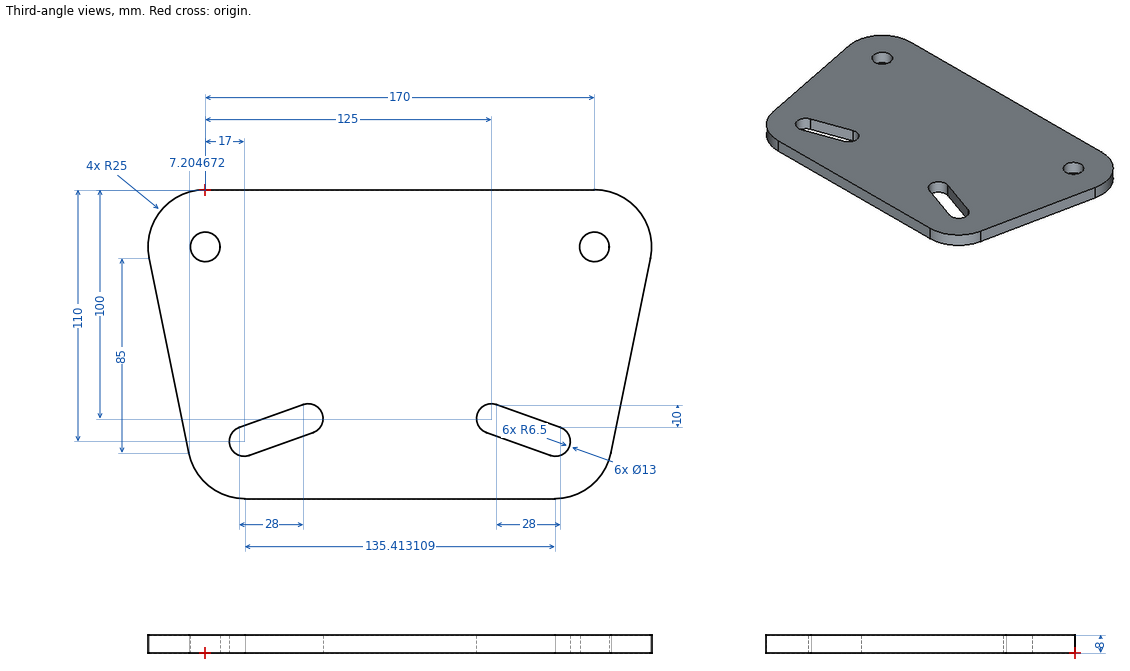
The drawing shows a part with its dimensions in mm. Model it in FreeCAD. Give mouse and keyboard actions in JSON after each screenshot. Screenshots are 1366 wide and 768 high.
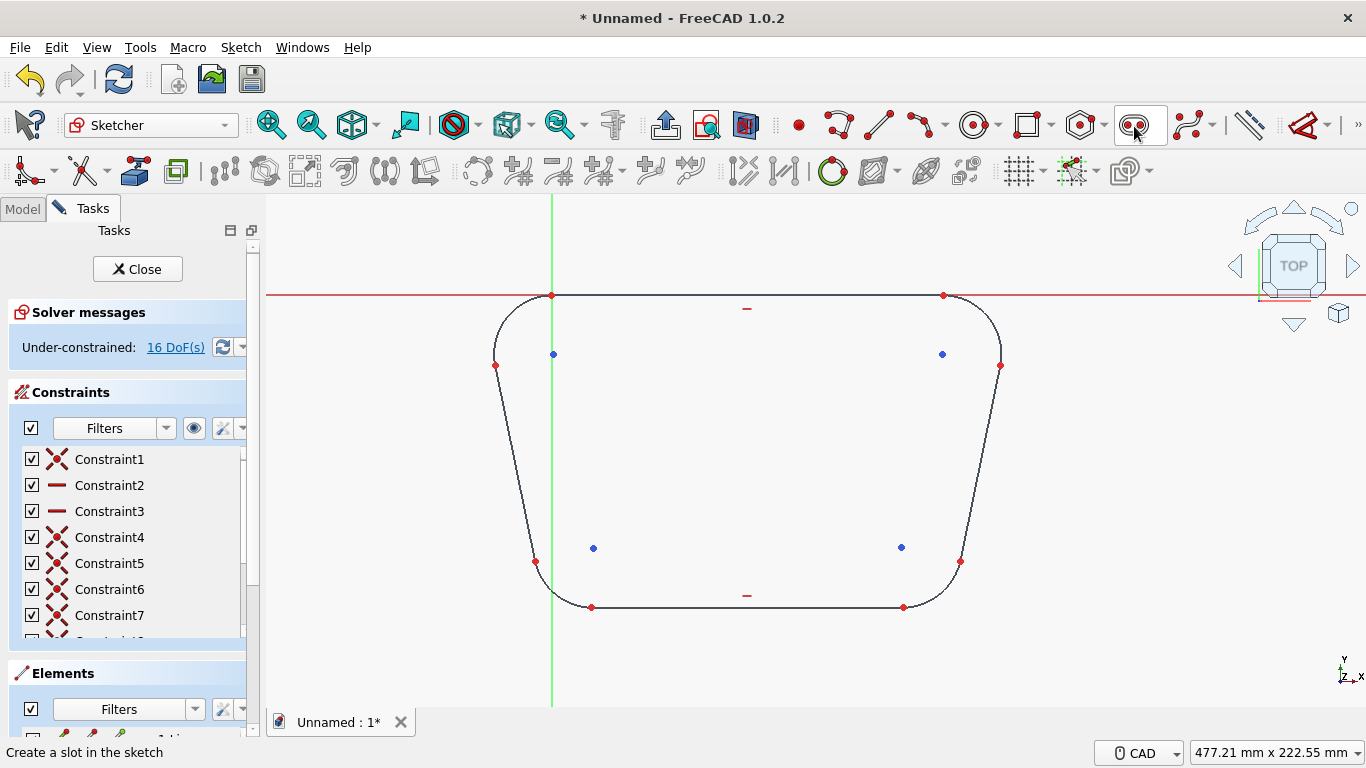
{"action": "scroll", "coordinate": [840, 526], "scroll_direction": "up", "scroll_amount": 3}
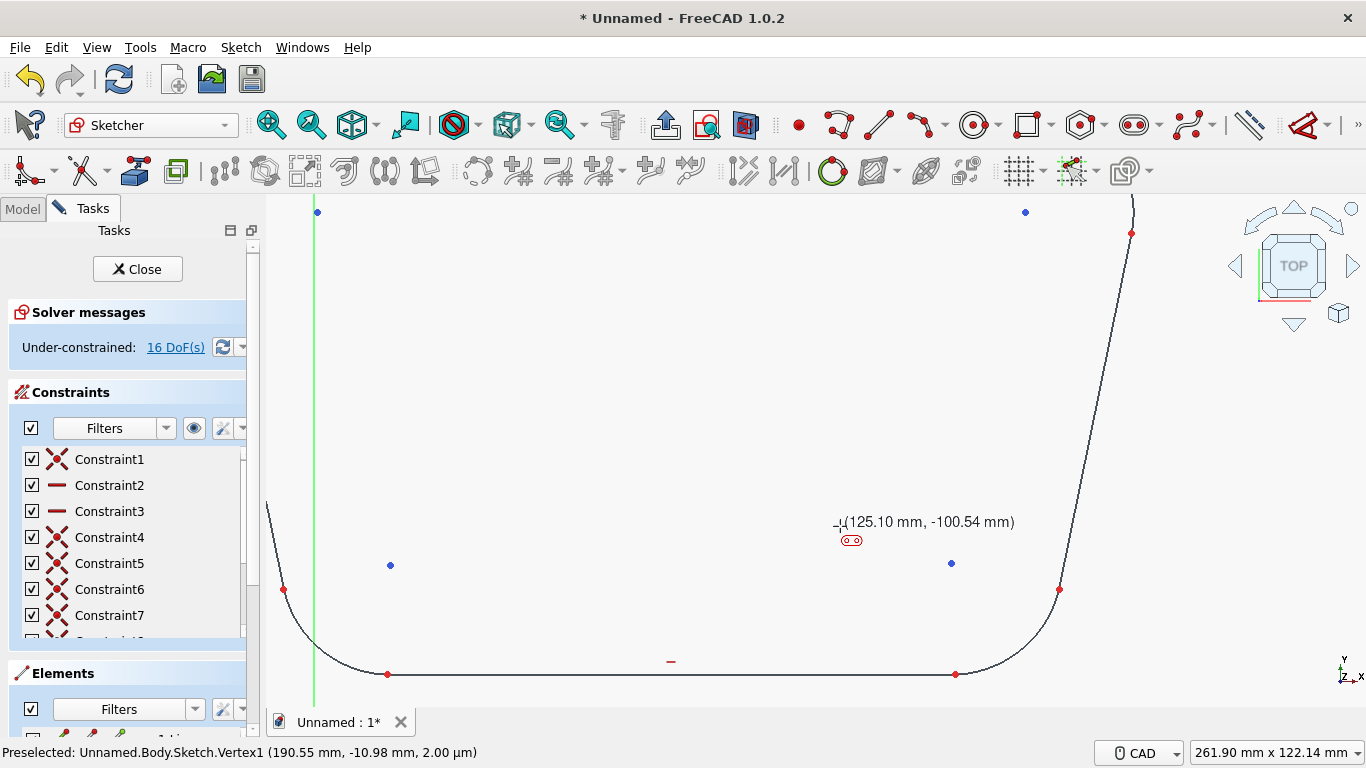
{"action": "left_click", "coordinate": [839, 525]}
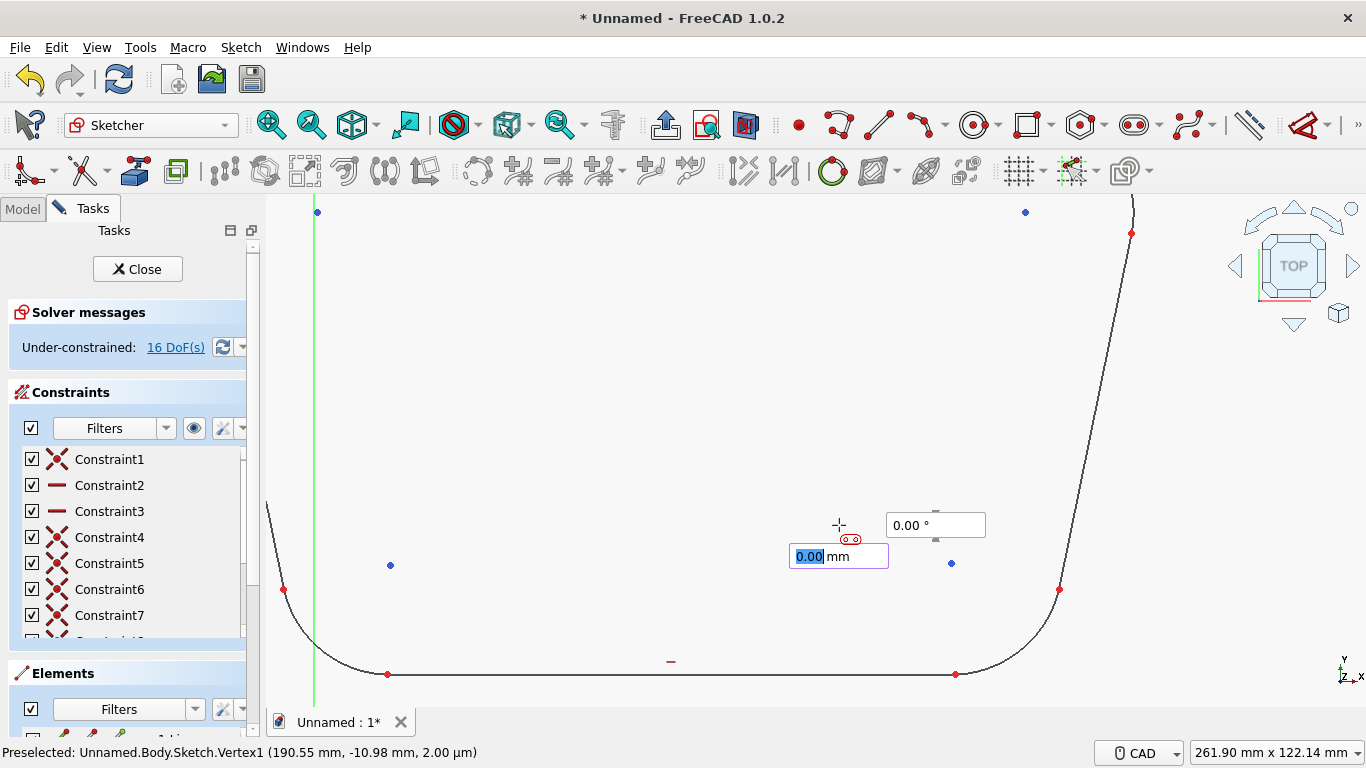
{"action": "scroll", "coordinate": [957, 567], "scroll_direction": "up", "scroll_amount": 13}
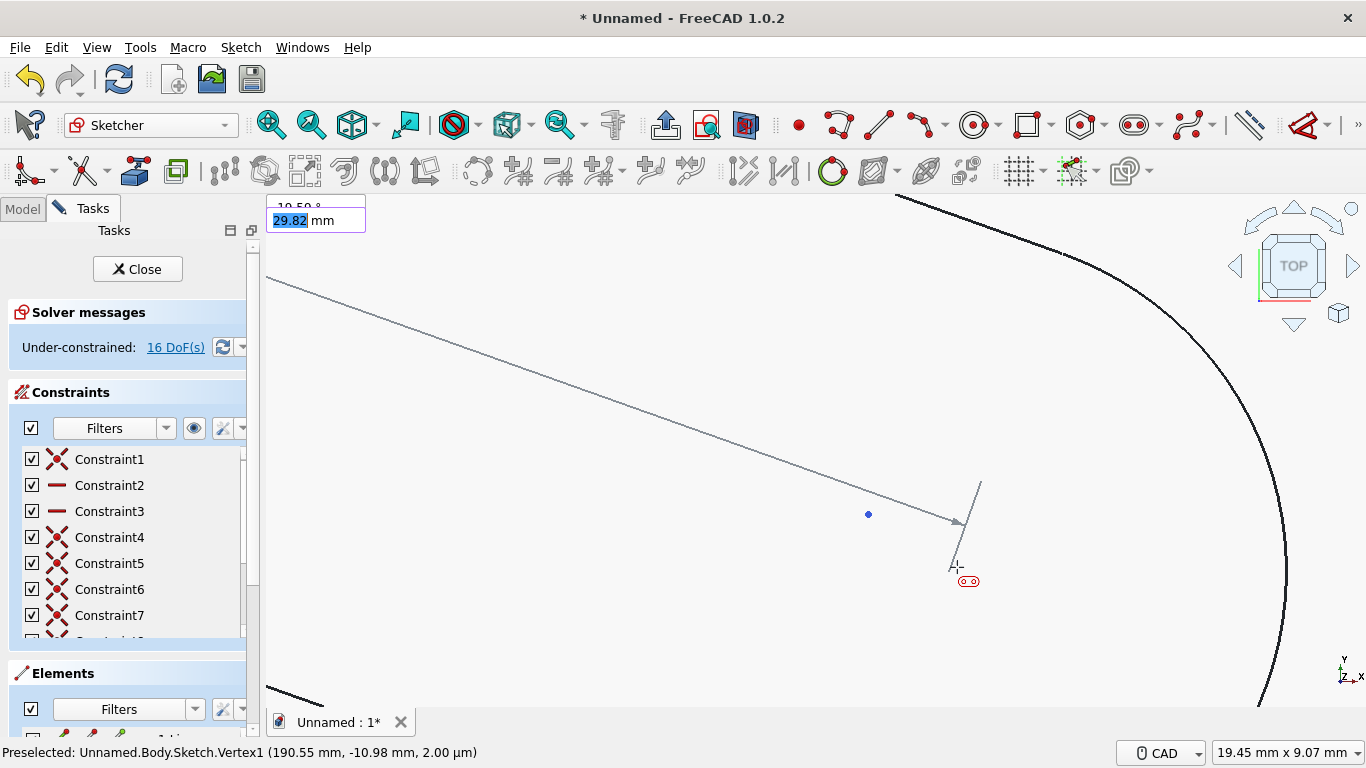
{"action": "left_click", "coordinate": [946, 558]}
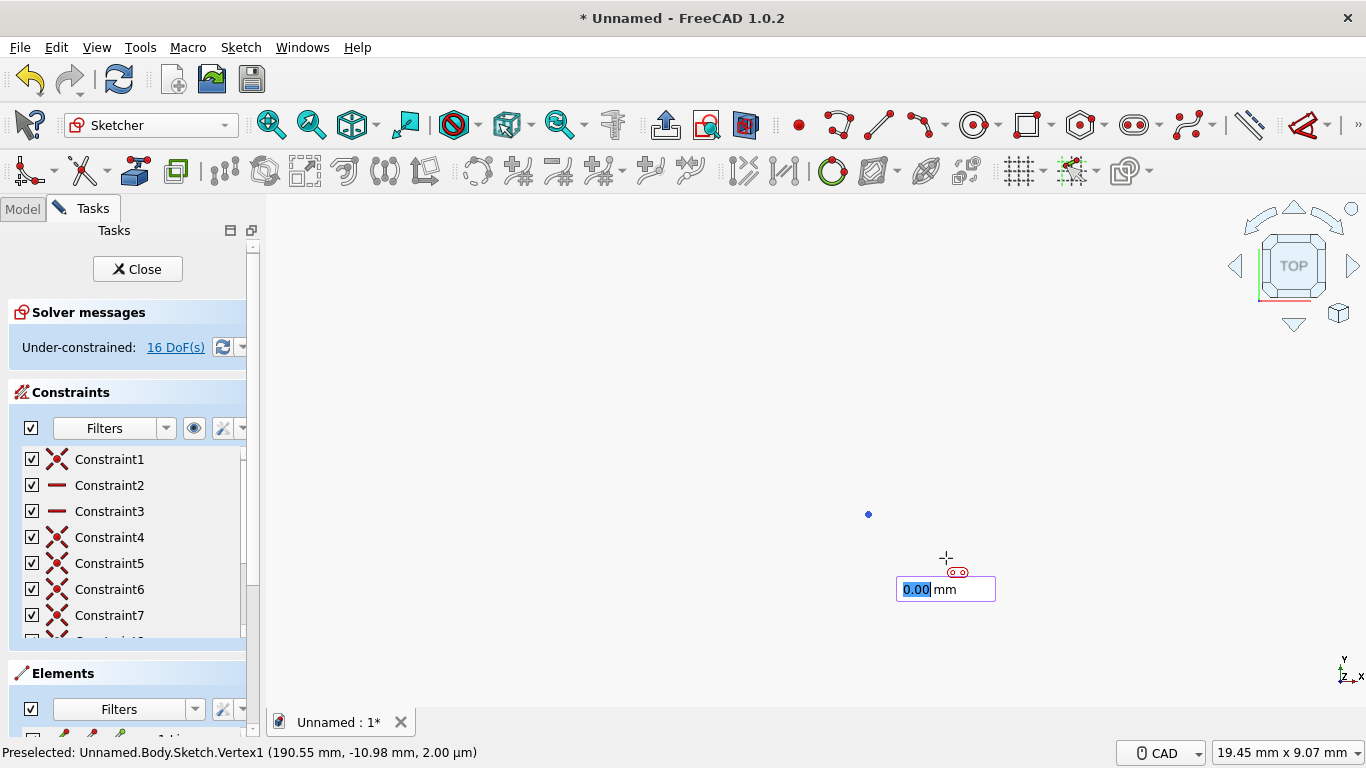
{"action": "scroll", "coordinate": [939, 571], "scroll_direction": "down", "scroll_amount": 15}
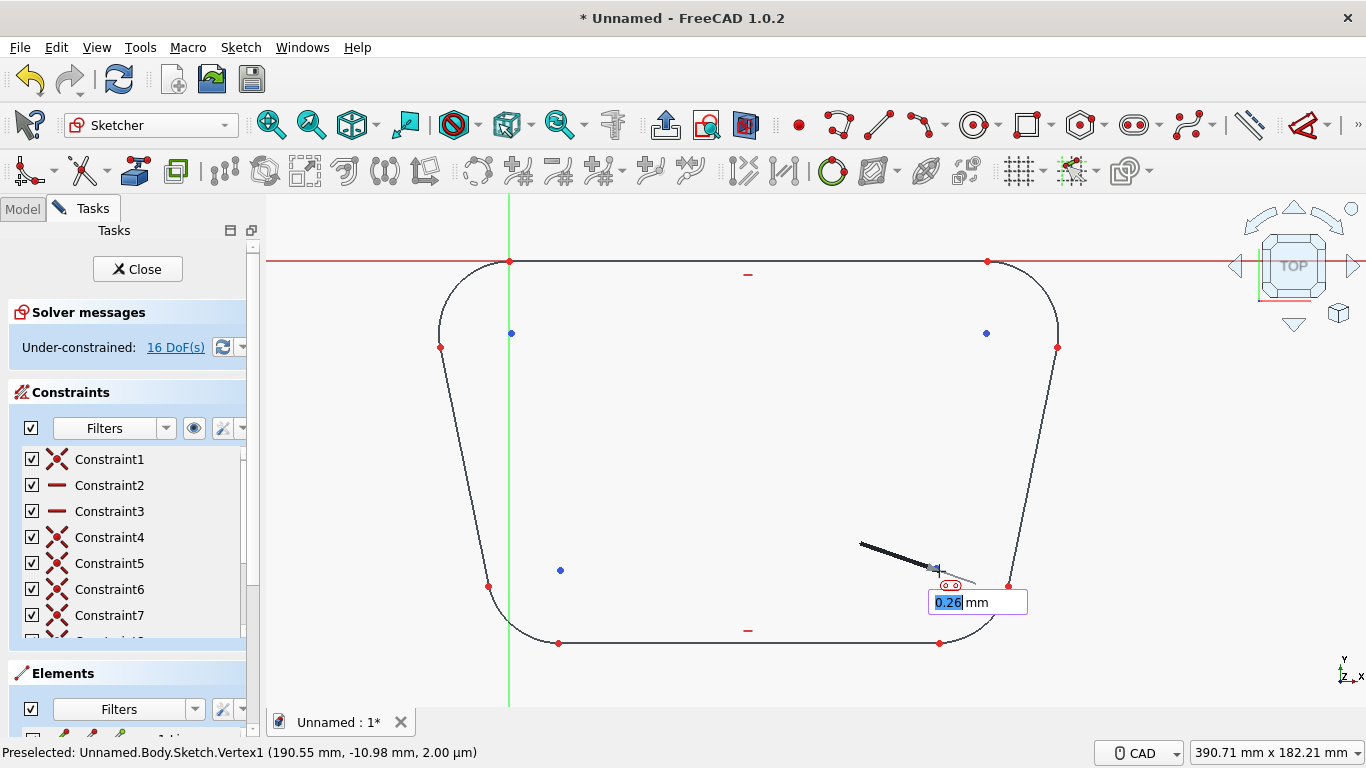
{"action": "left_click", "coordinate": [907, 540]}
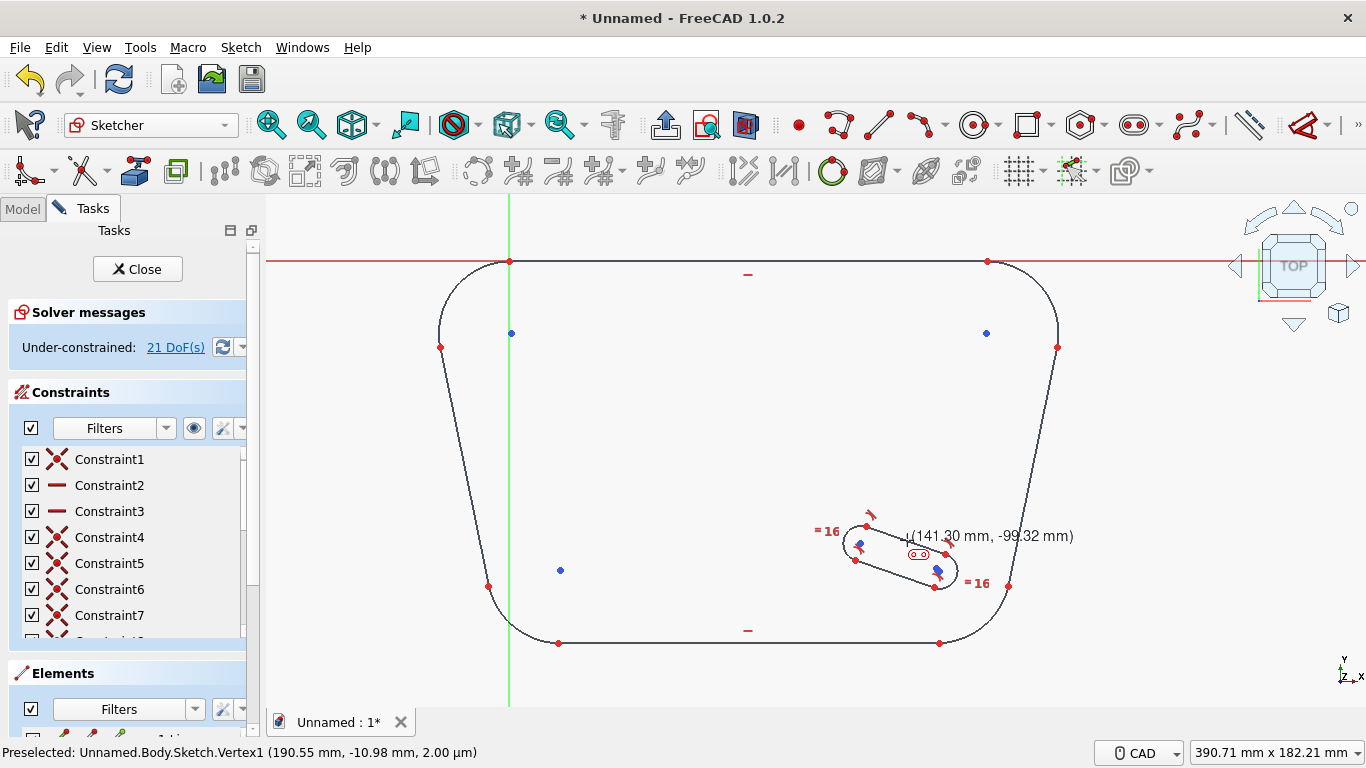
{"action": "scroll", "coordinate": [557, 571], "scroll_direction": "up", "scroll_amount": 15}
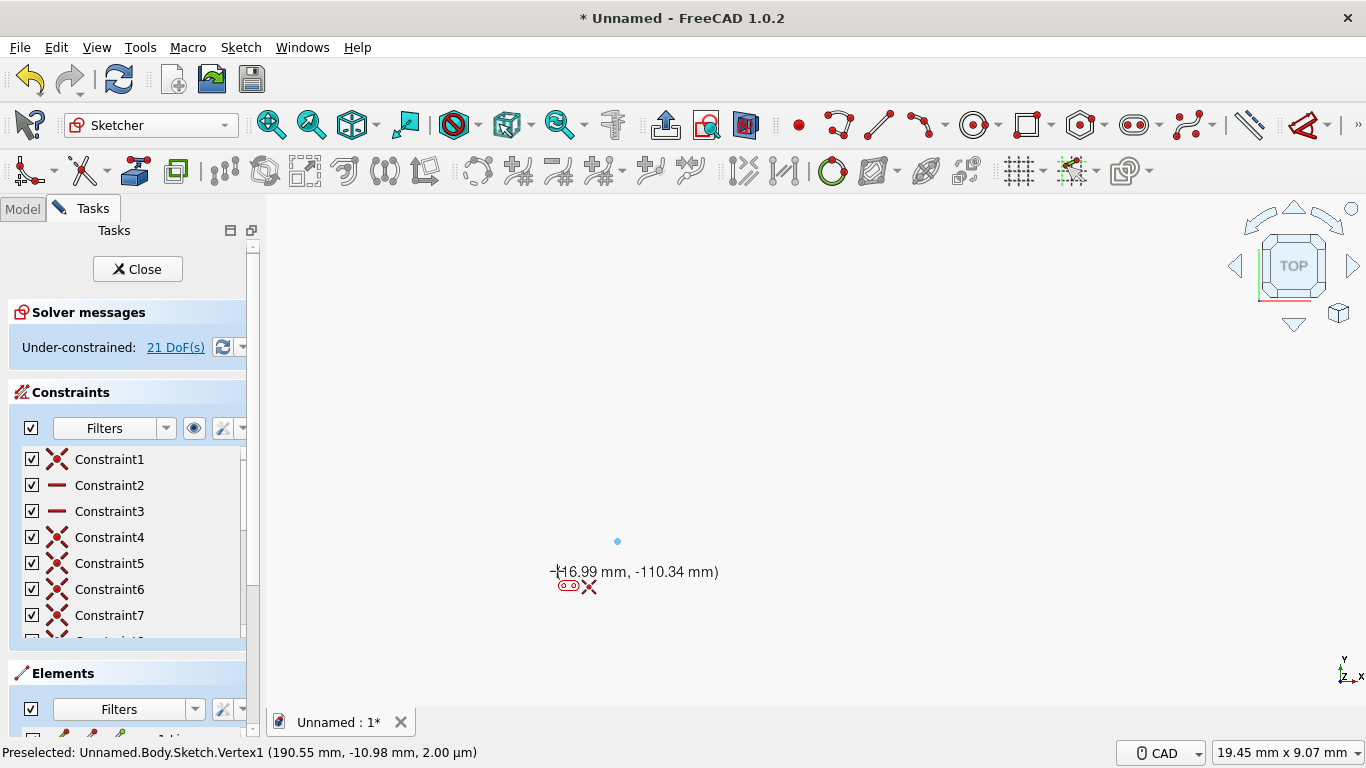
{"action": "left_click", "coordinate": [553, 558]}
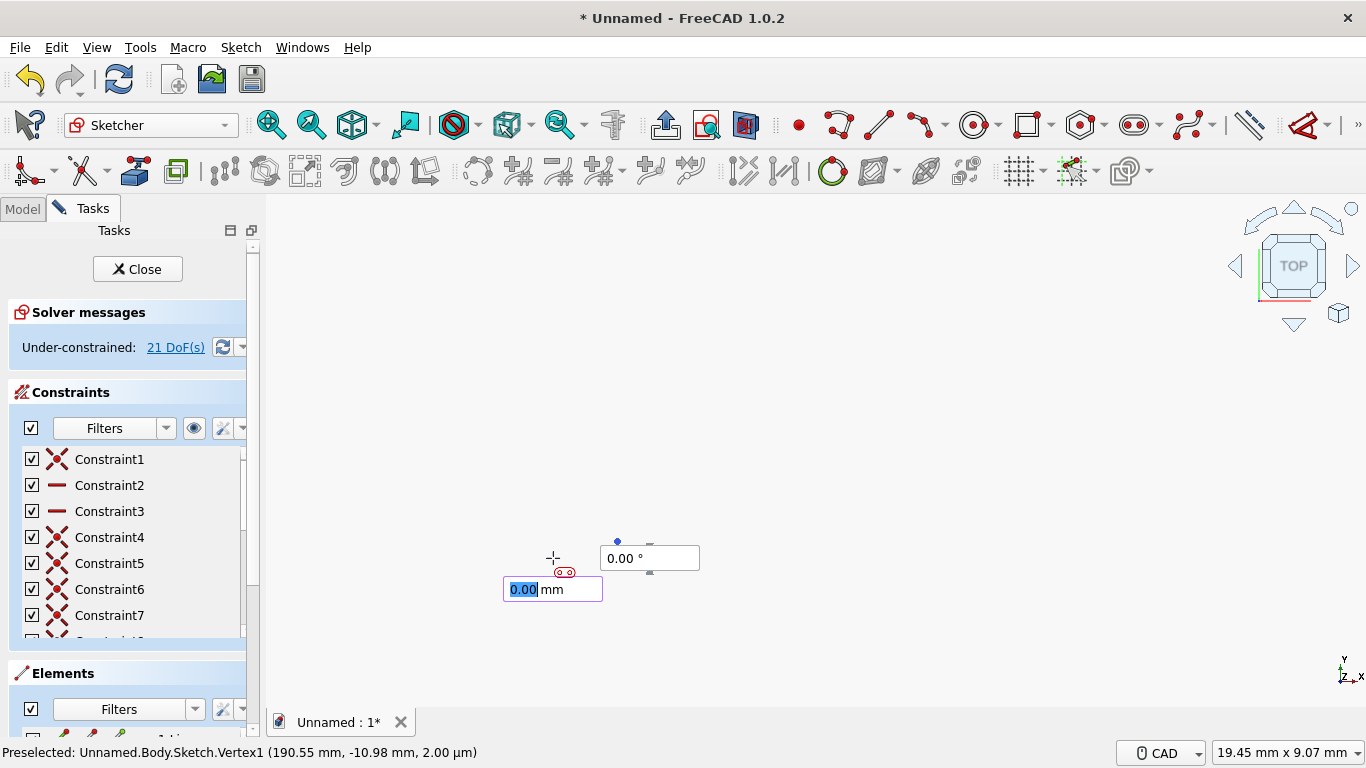
{"action": "scroll", "coordinate": [556, 571], "scroll_direction": "down", "scroll_amount": 15}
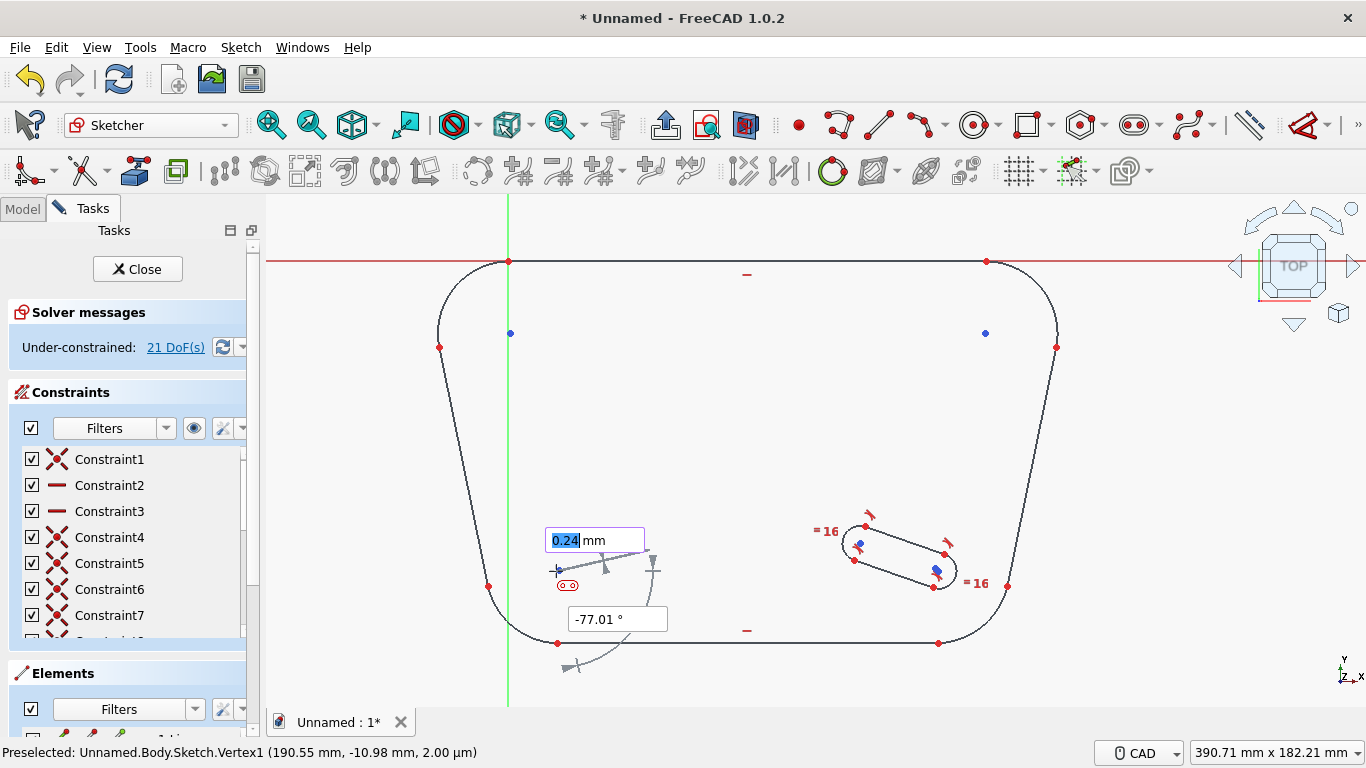
{"action": "left_click", "coordinate": [635, 543]}